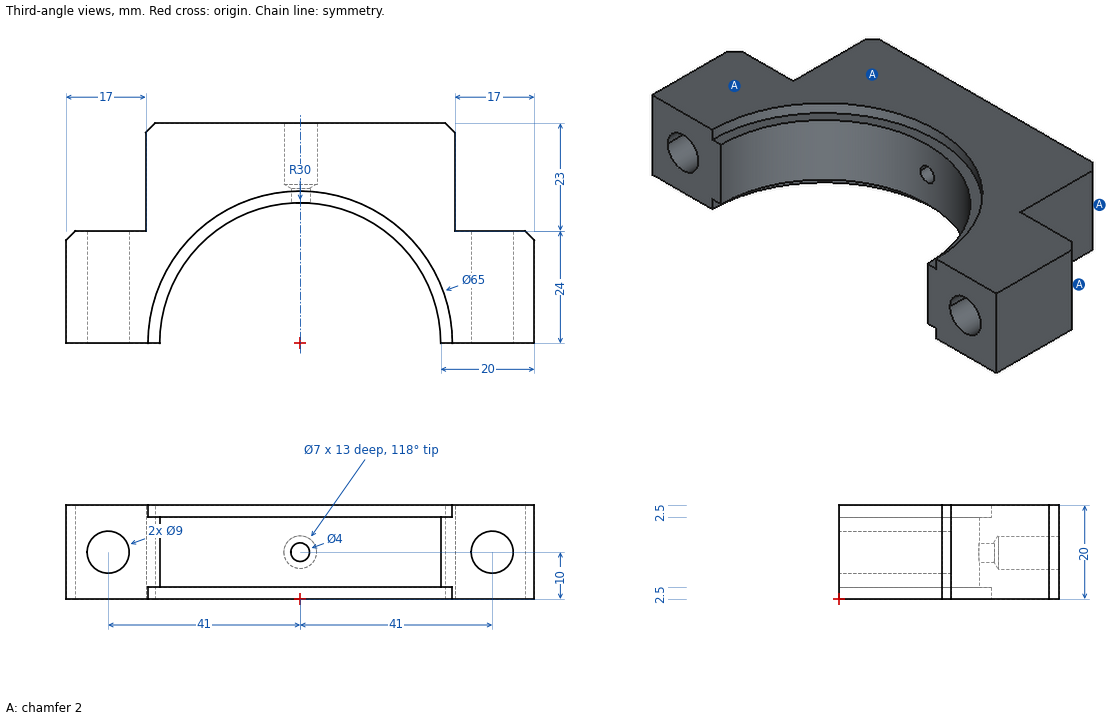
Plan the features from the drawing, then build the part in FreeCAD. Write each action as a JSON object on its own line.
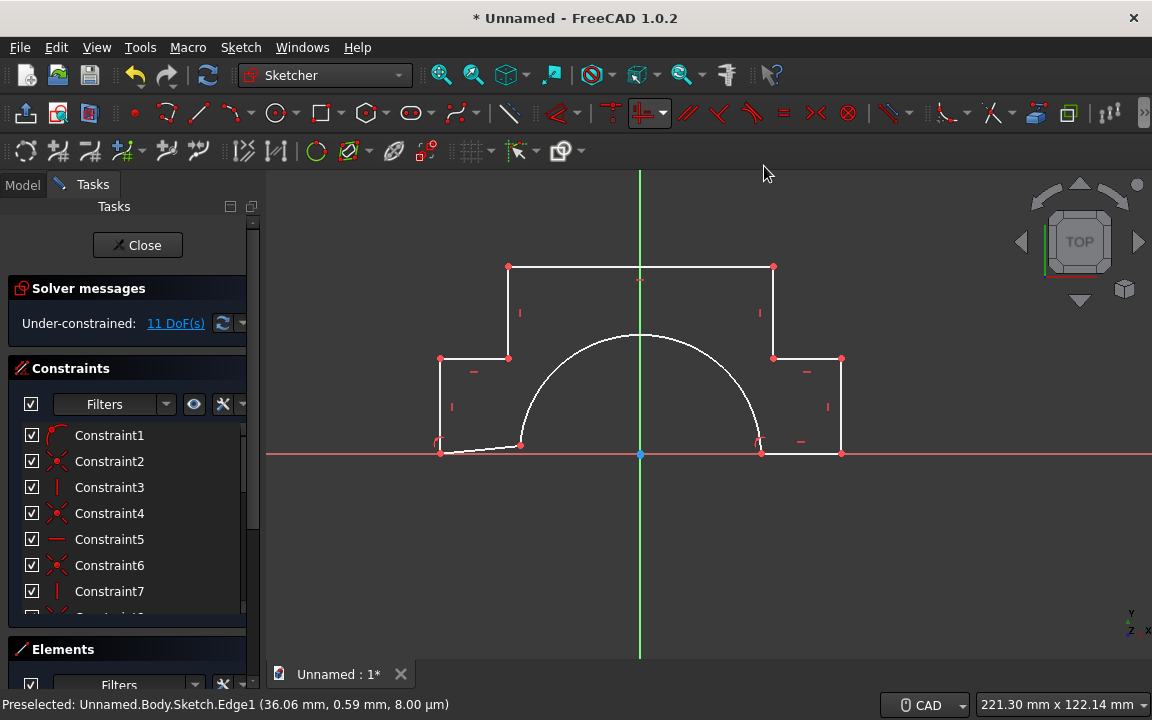
{"action": "left_click", "coordinate": [464, 452]}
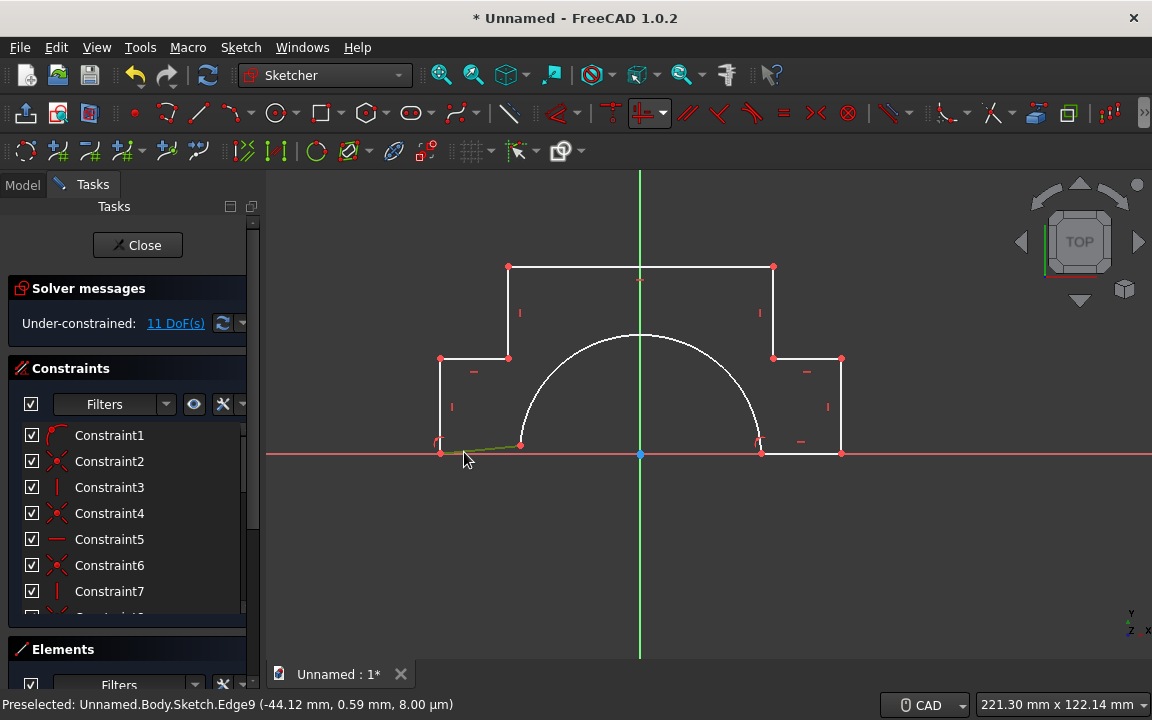
{"action": "key", "text": "h"}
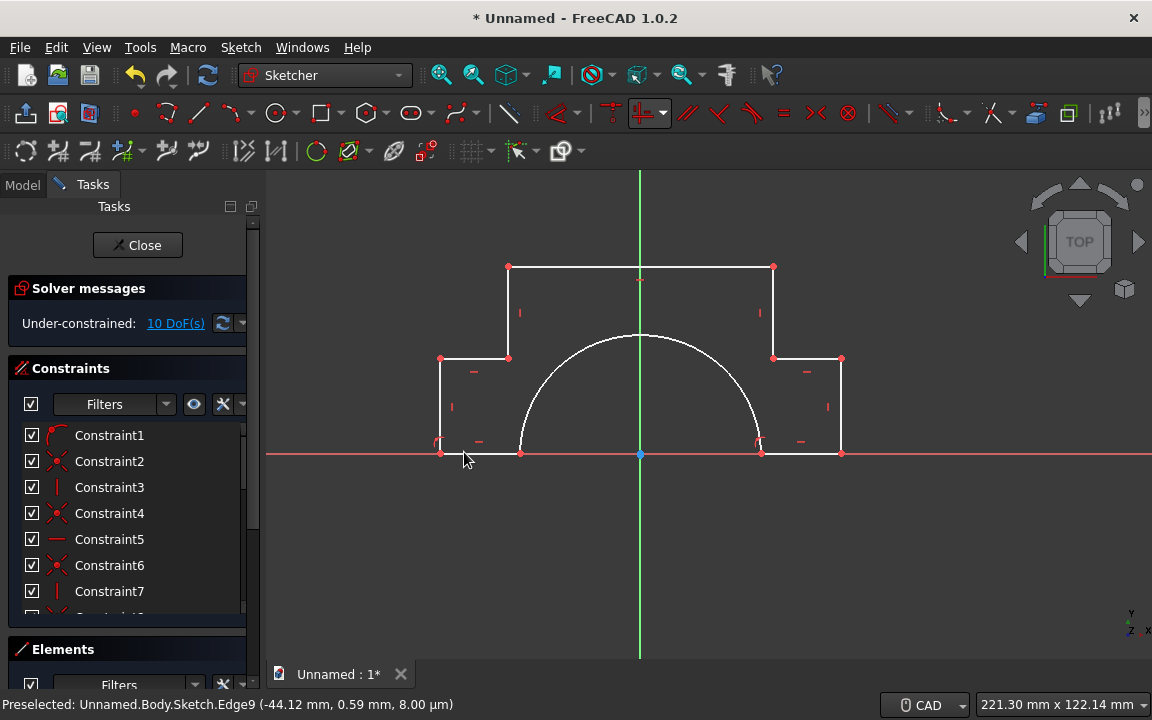
{"action": "left_click_drag", "start_coordinate": [630, 444], "coordinate": [650, 466]}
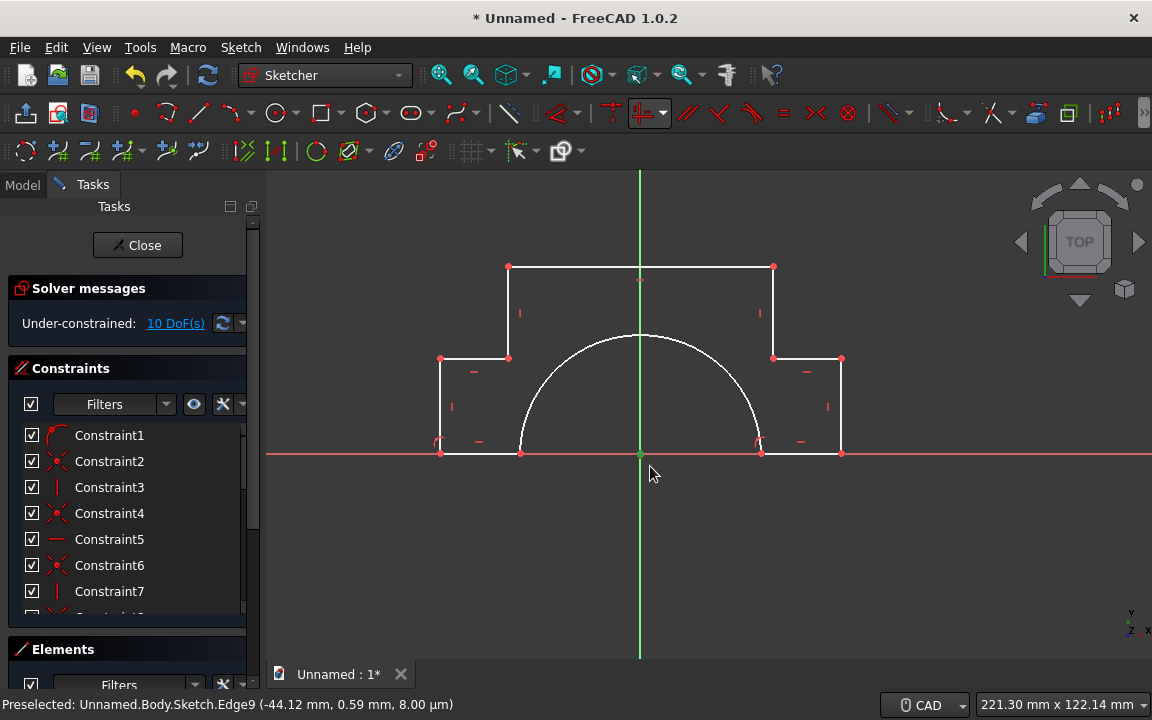
{"action": "left_click", "coordinate": [612, 114]}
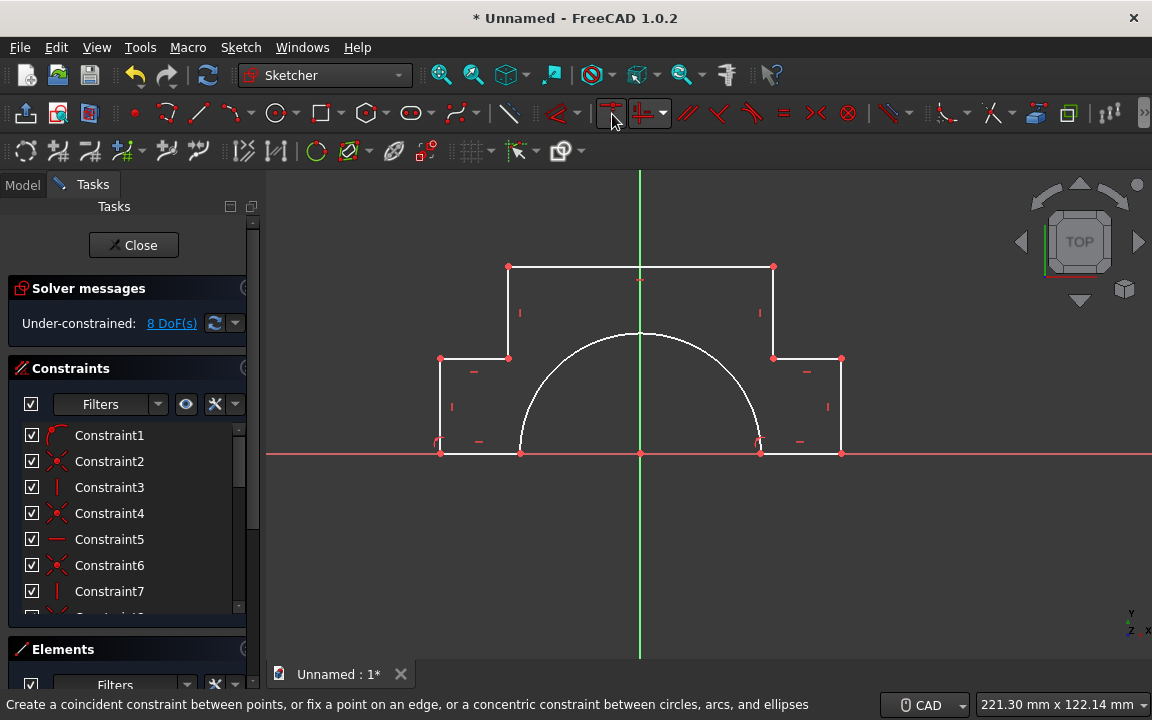
{"action": "left_click", "coordinate": [773, 359]}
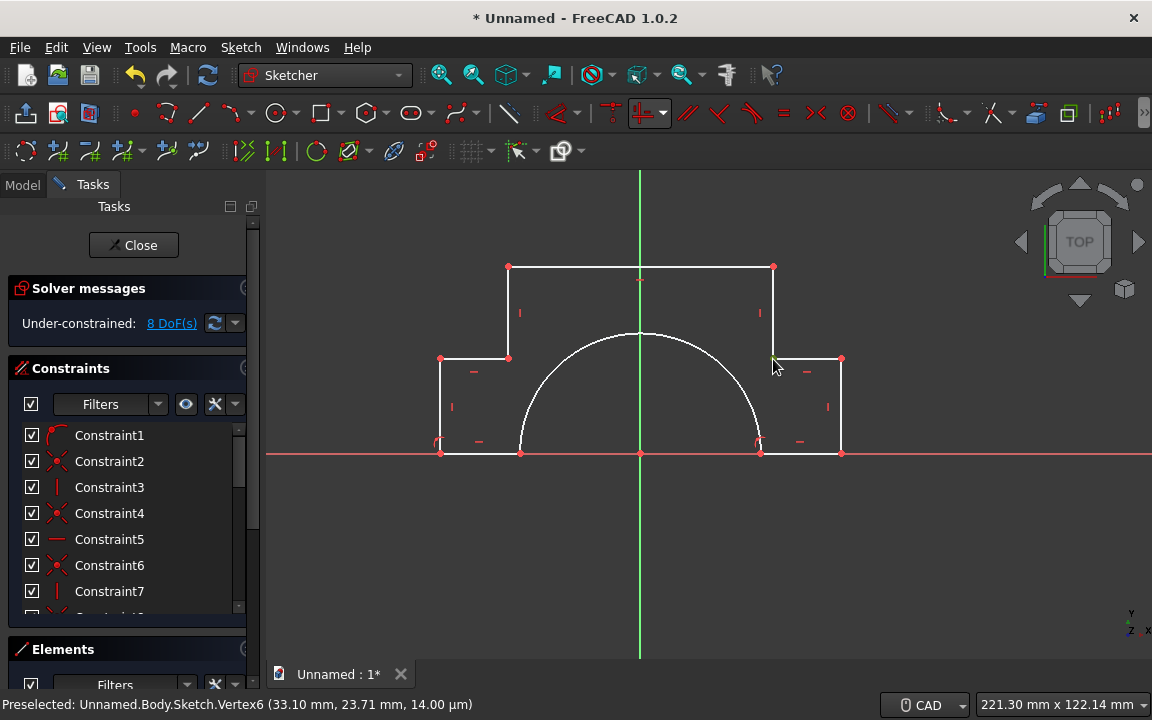
{"action": "left_click", "coordinate": [508, 359]}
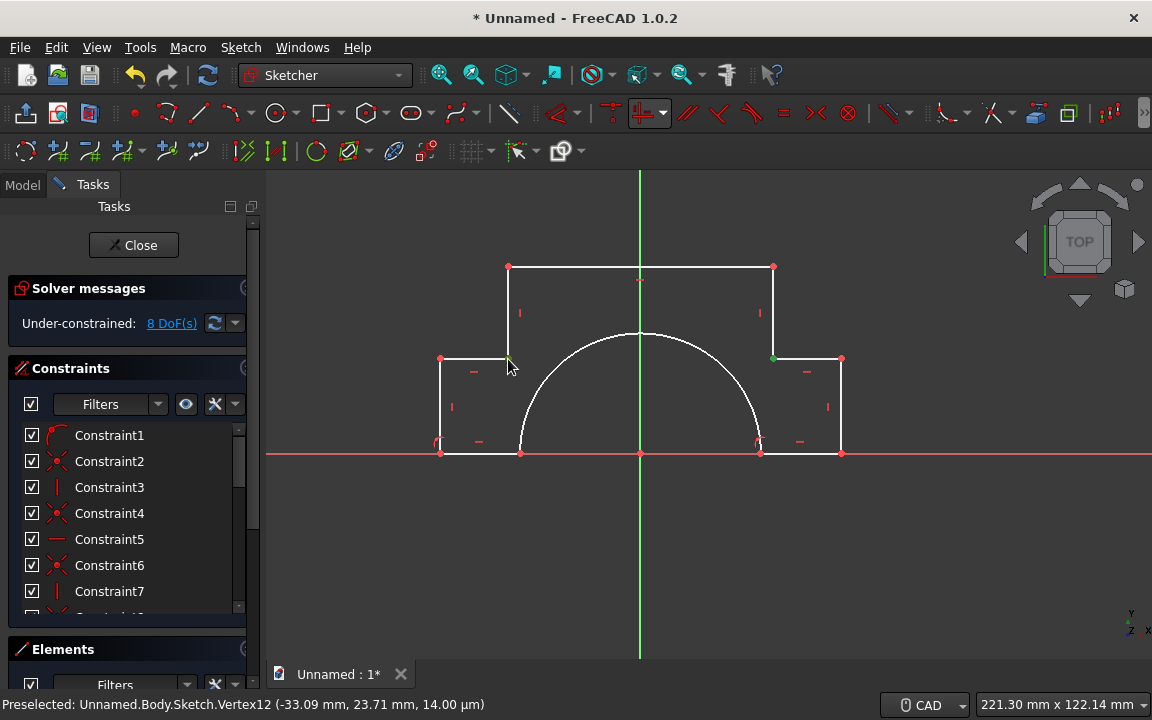
{"action": "left_click", "coordinate": [640, 600]}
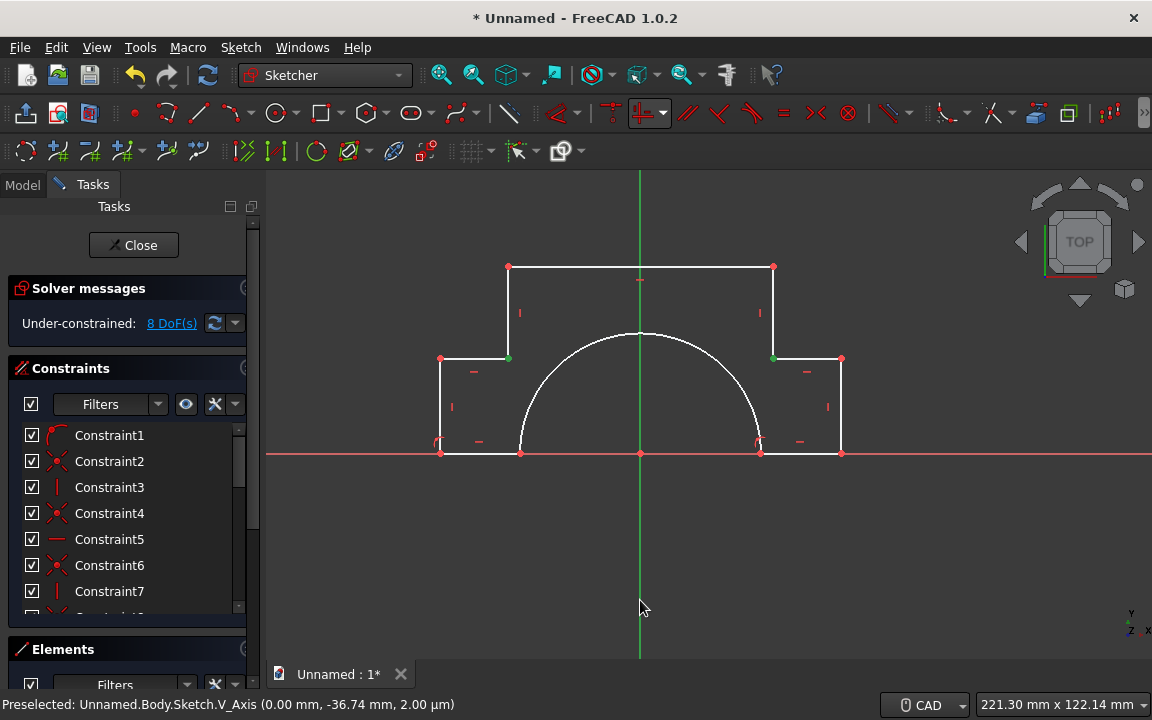
{"action": "left_click", "coordinate": [816, 114]}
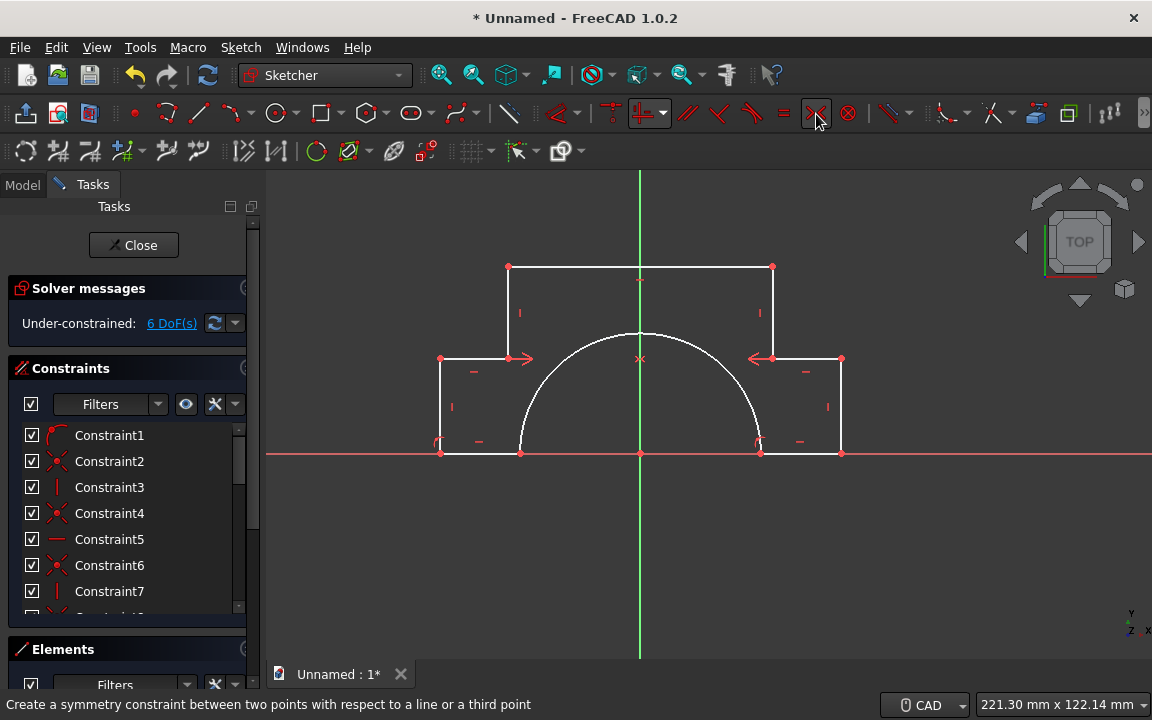
{"action": "left_click", "coordinate": [556, 114]}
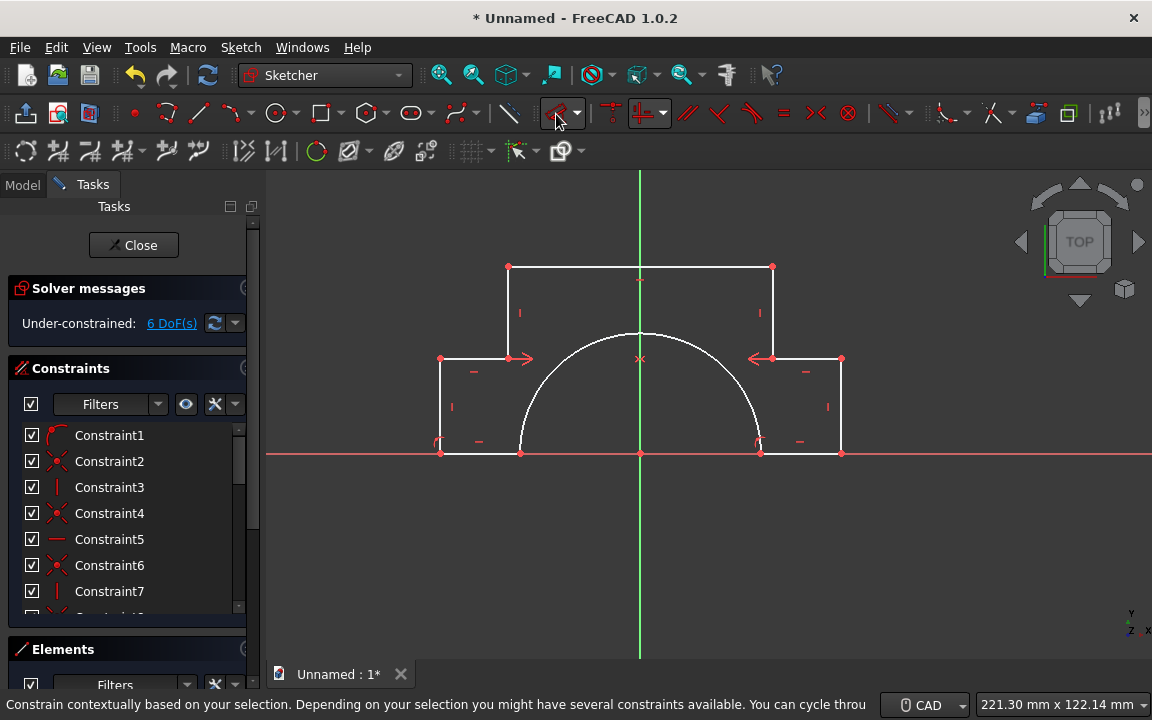
{"action": "left_click", "coordinate": [711, 356]}
{"action": "left_click", "coordinate": [730, 330]}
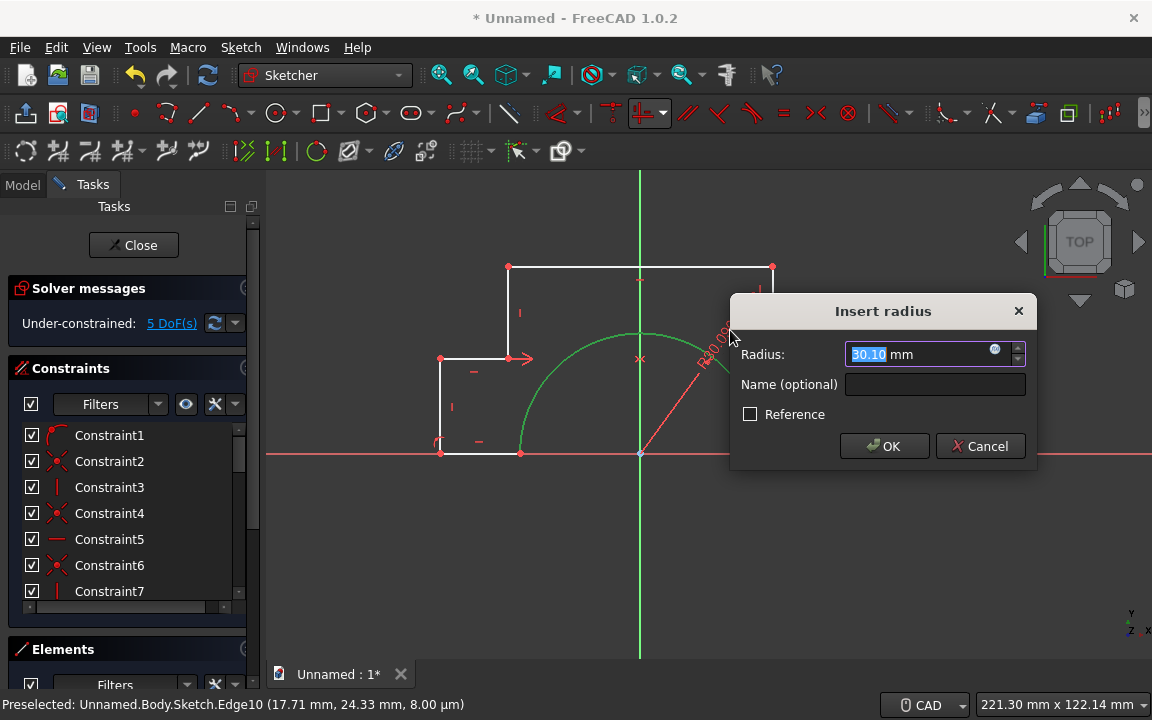
{"action": "type", "text": "30"}
{"action": "key", "text": "Return"}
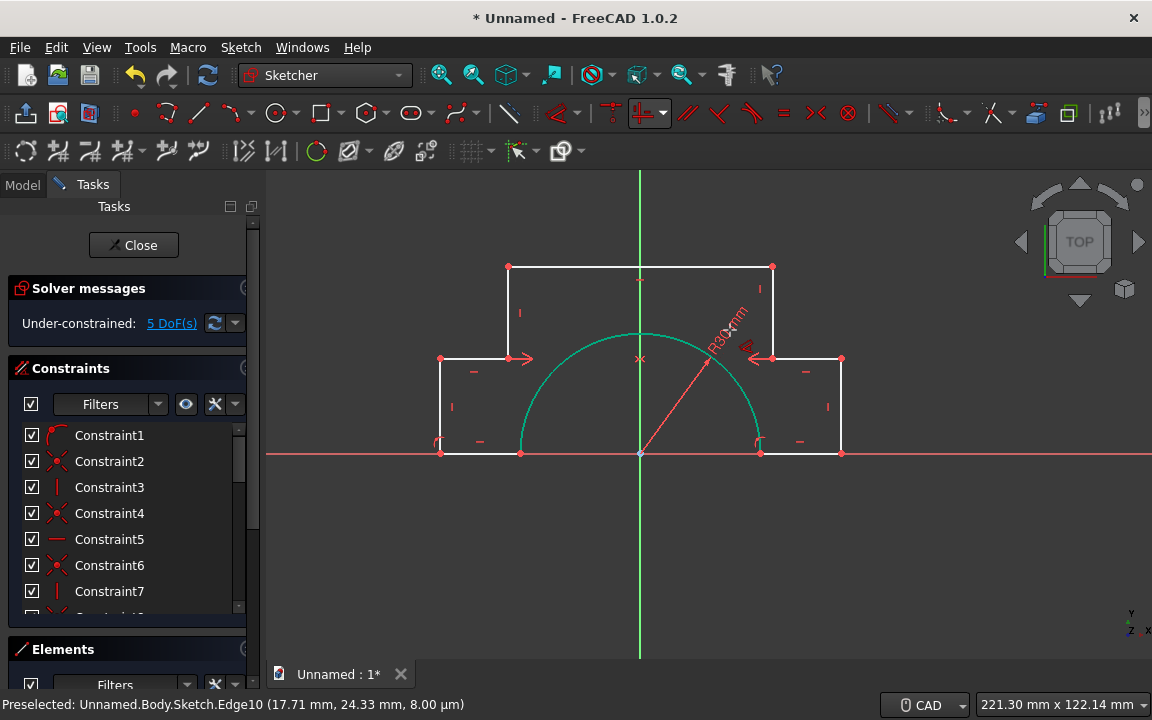
{"action": "left_click", "coordinate": [785, 454]}
{"action": "left_click", "coordinate": [801, 488]}